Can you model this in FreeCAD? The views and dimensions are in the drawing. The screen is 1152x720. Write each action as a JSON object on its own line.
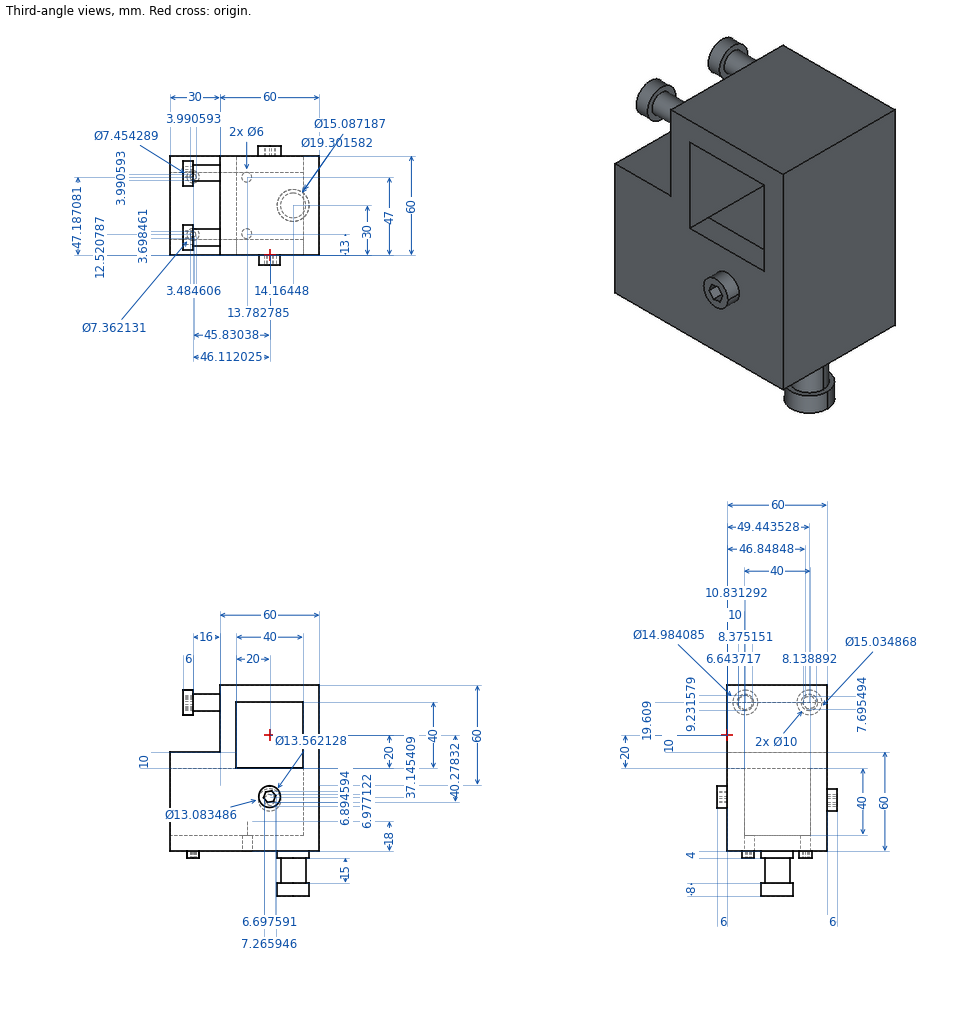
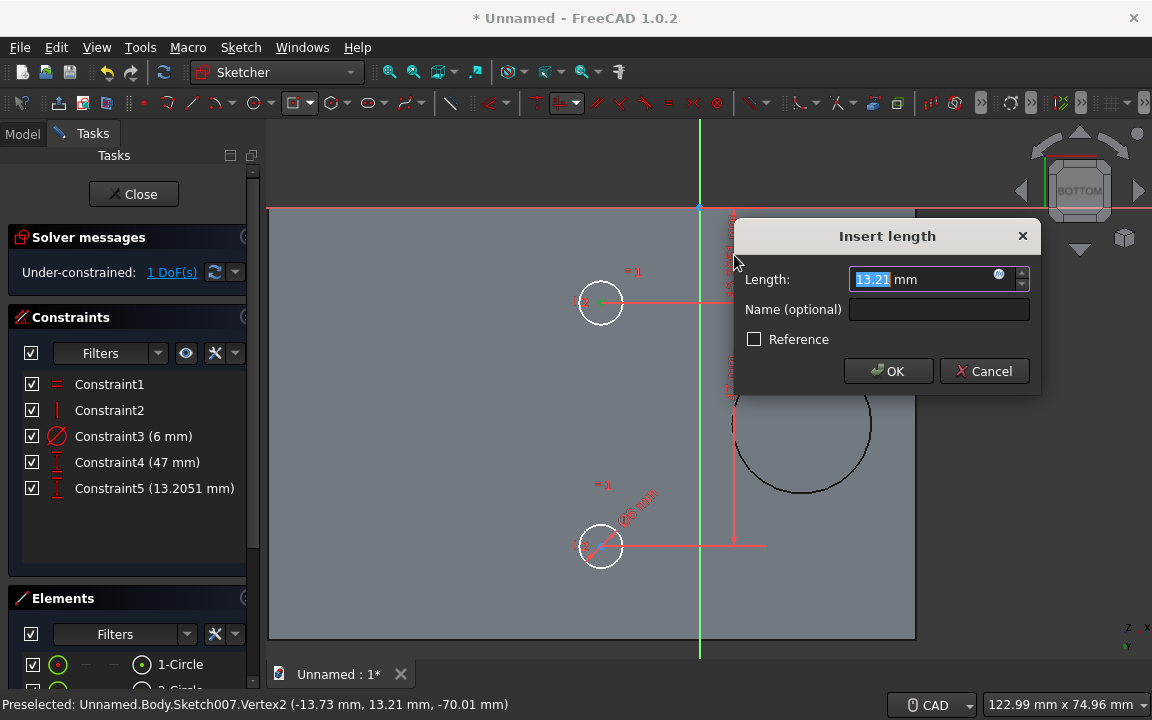
{"action": "type", "text": "13"}
{"action": "key", "text": "Return"}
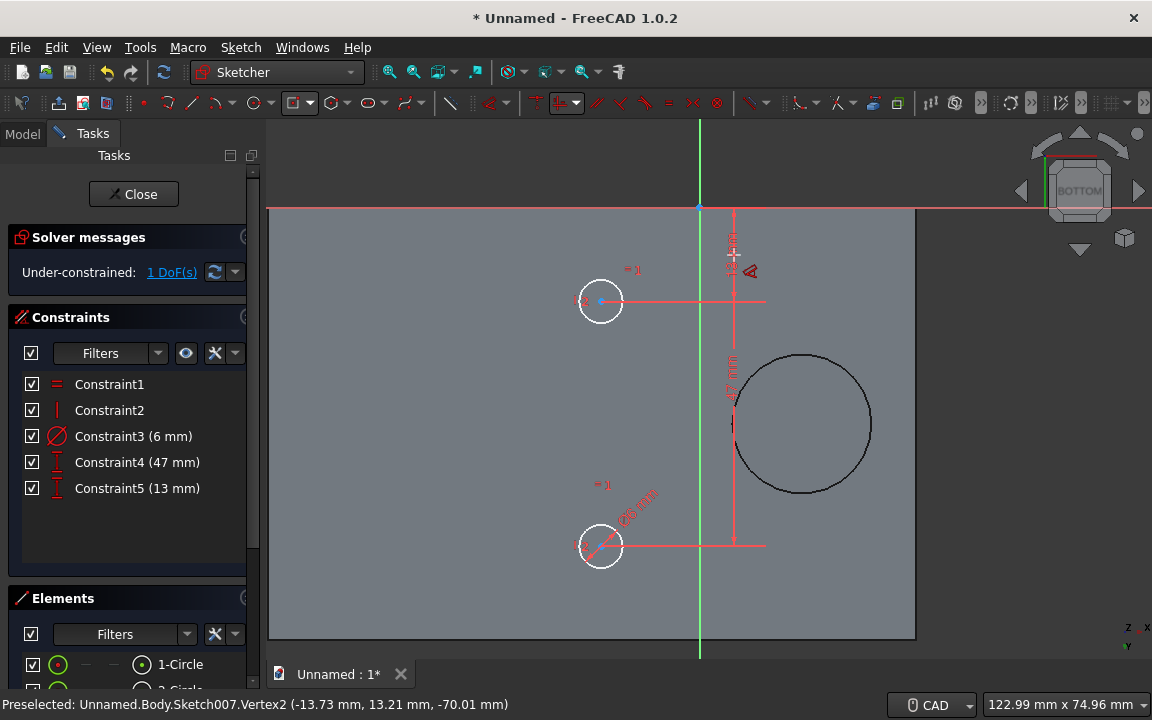
{"action": "left_click", "coordinate": [601, 546]}
{"action": "left_click", "coordinate": [650, 174]}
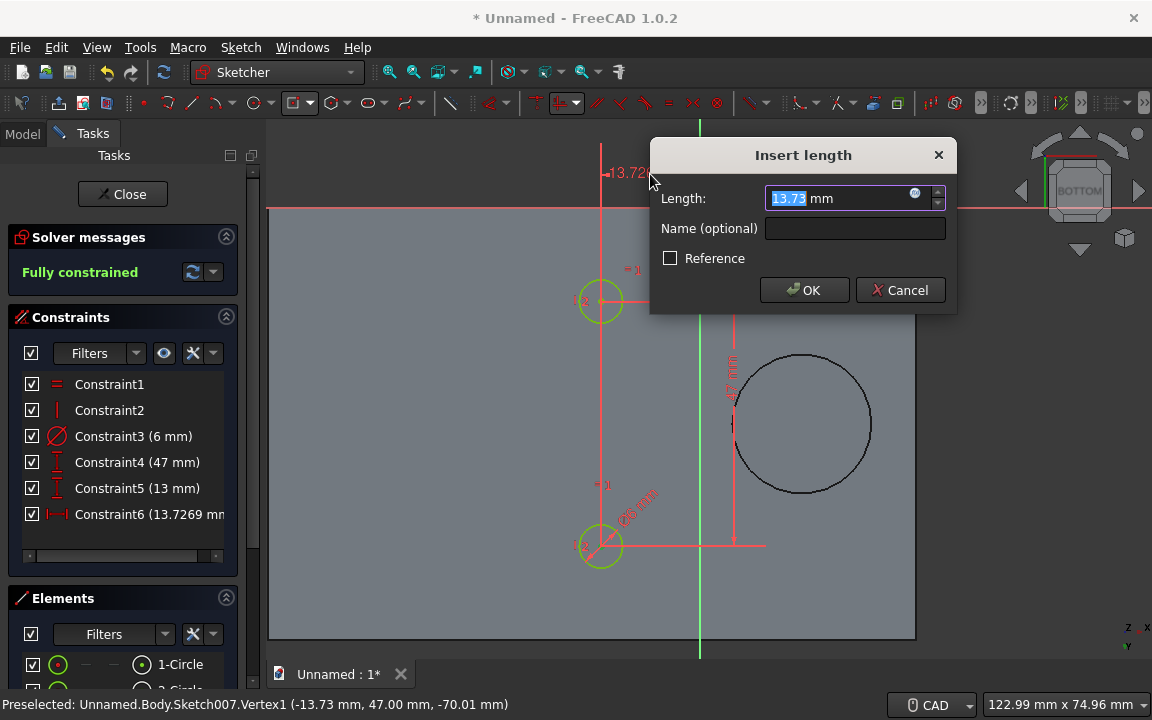
{"action": "type", "text": "13.782785"}
{"action": "key", "text": "Return"}
{"action": "key", "text": "Escape"}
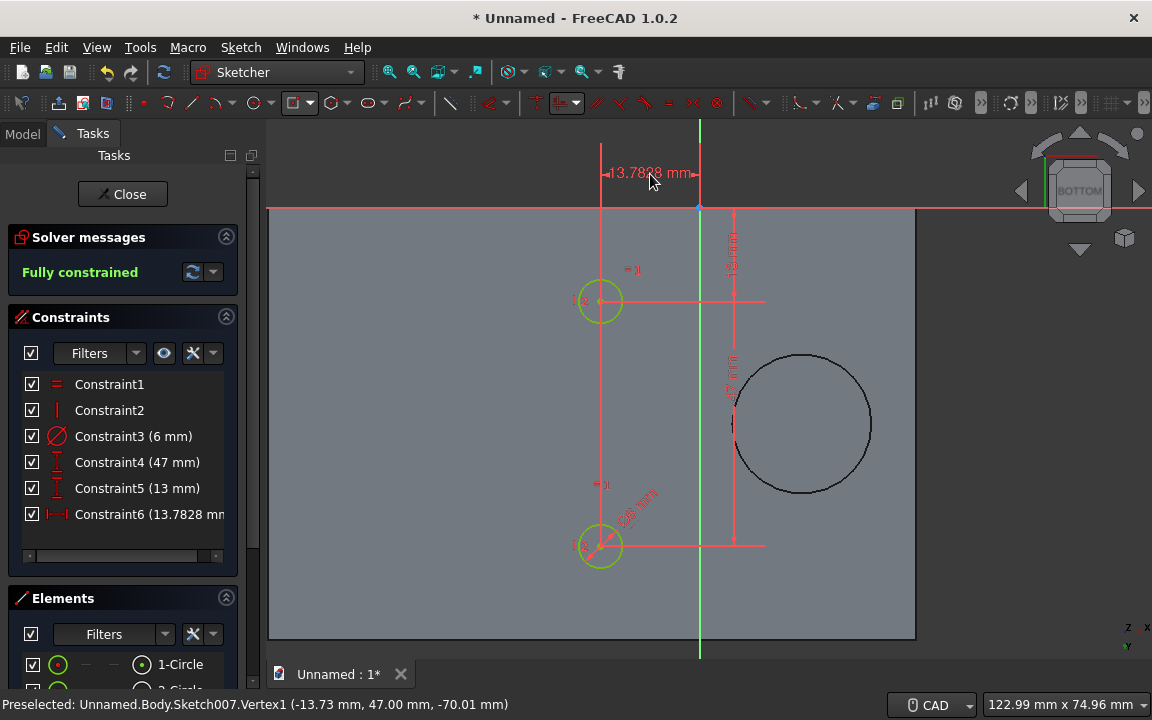
{"action": "left_click", "coordinate": [123, 194]}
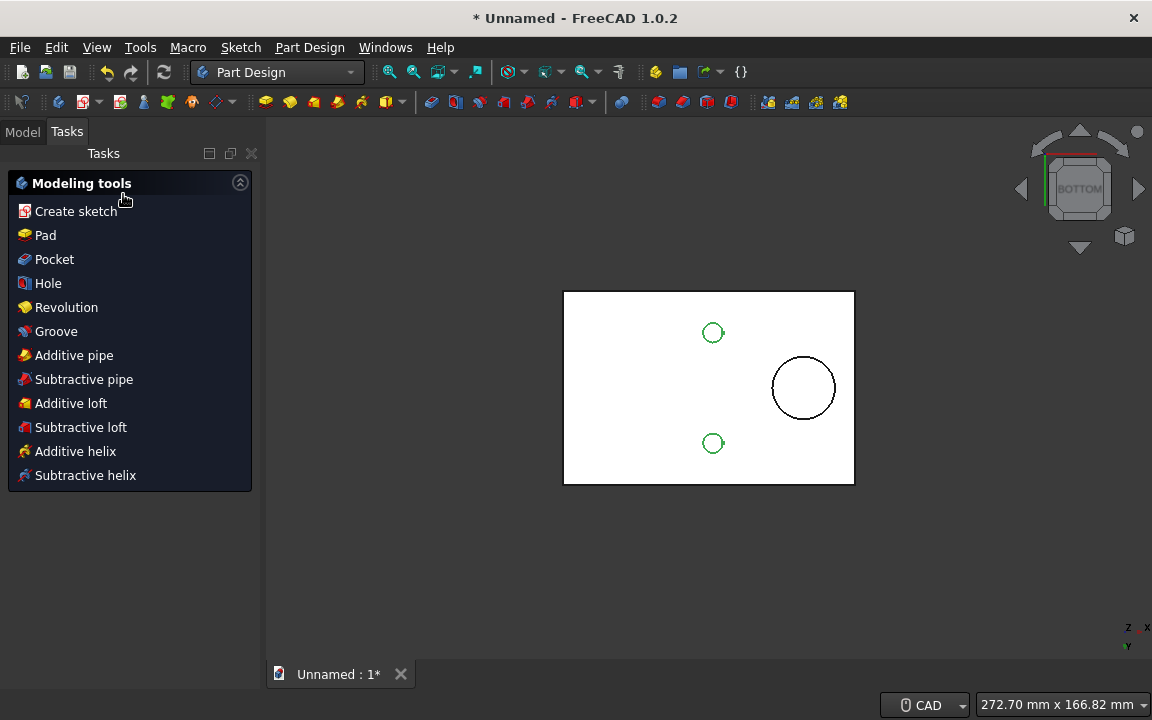
{"action": "left_click", "coordinate": [432, 102]}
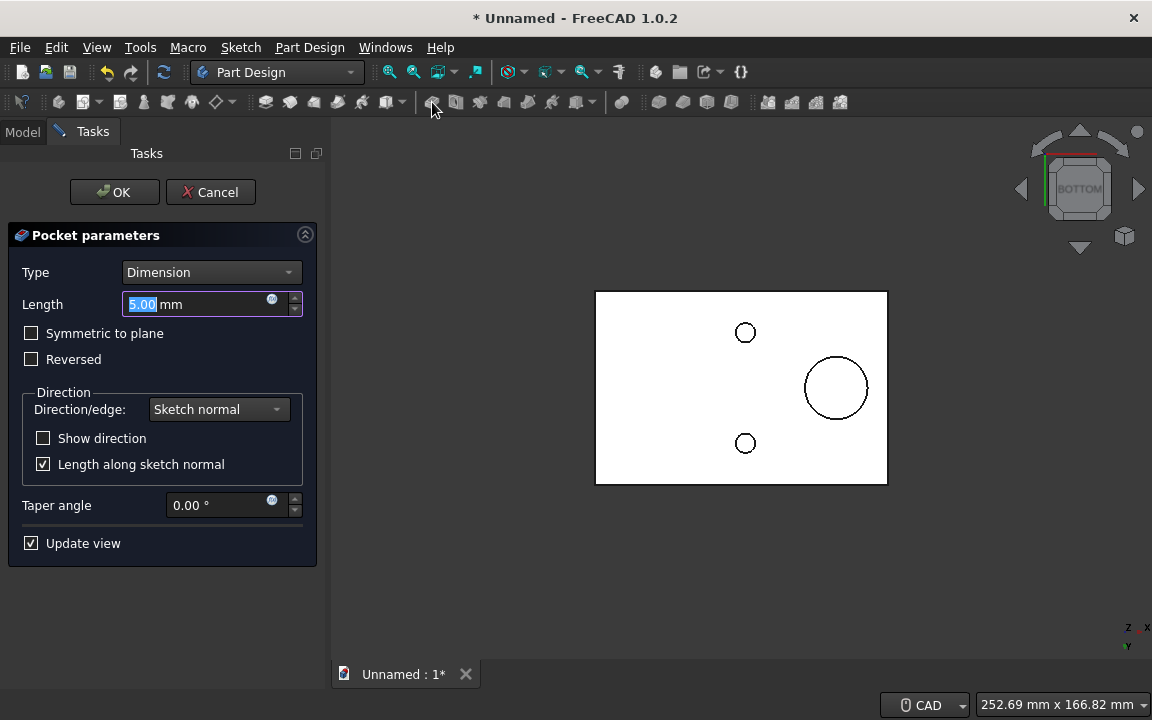
{"action": "type", "text": "18"}
{"action": "key", "text": "Tab"}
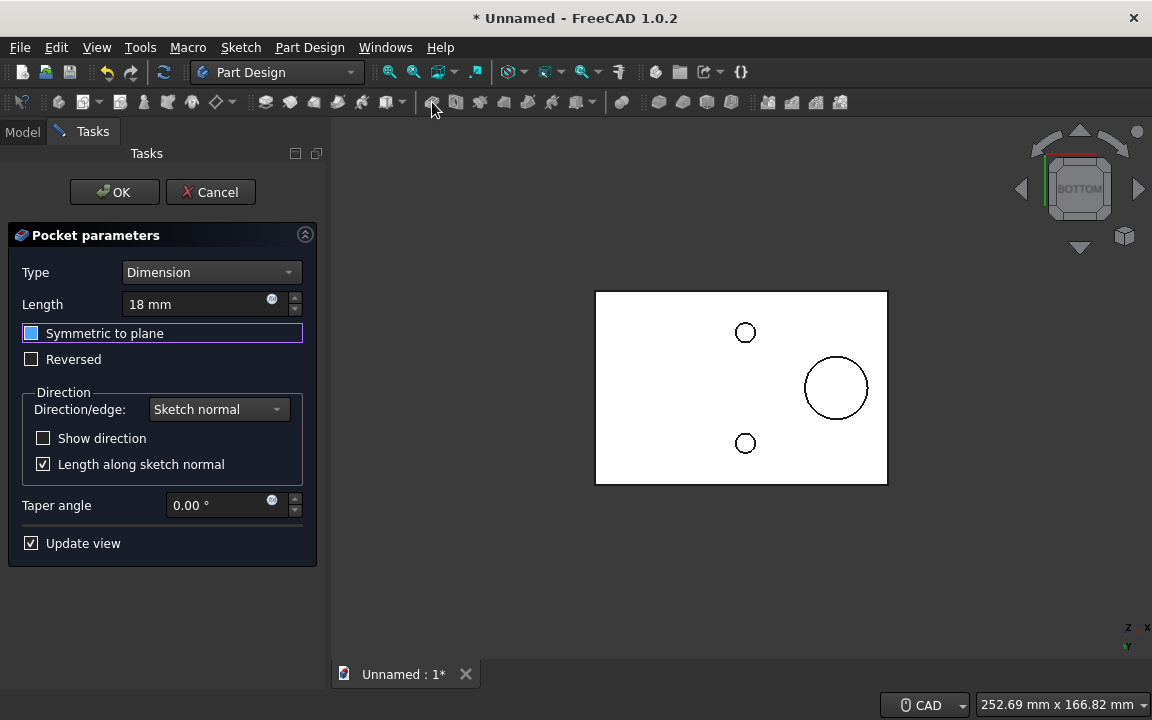
{"action": "left_click", "coordinate": [115, 192]}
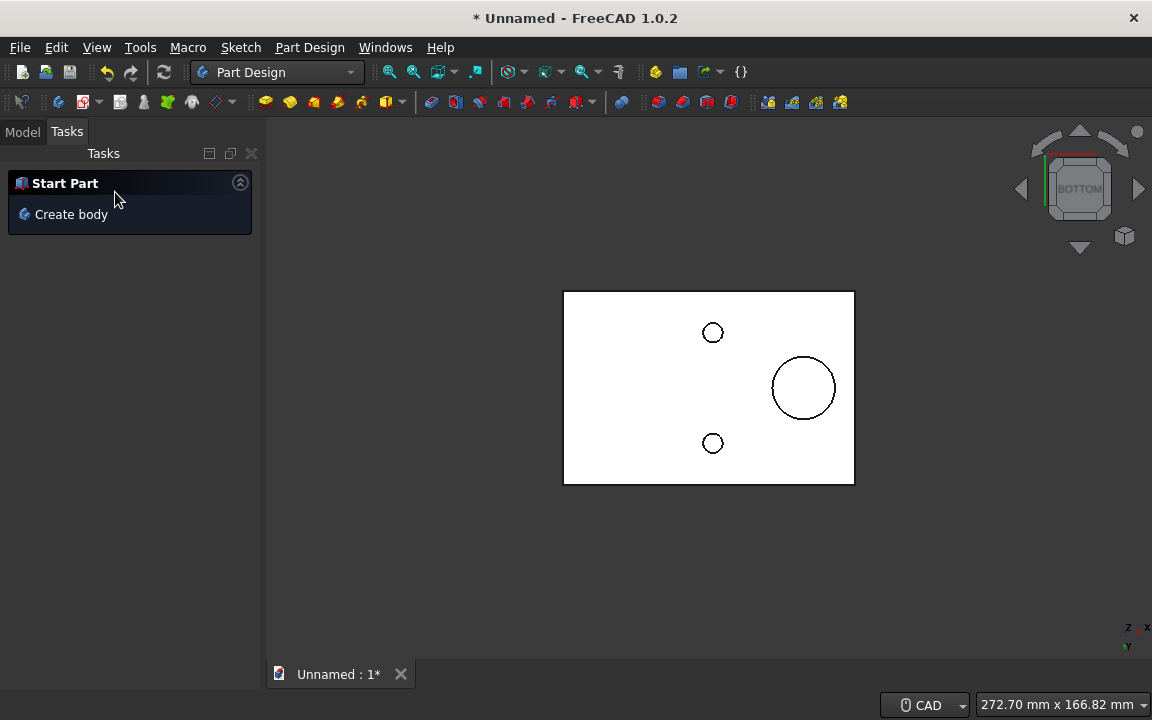
{"action": "left_click", "coordinate": [390, 72]}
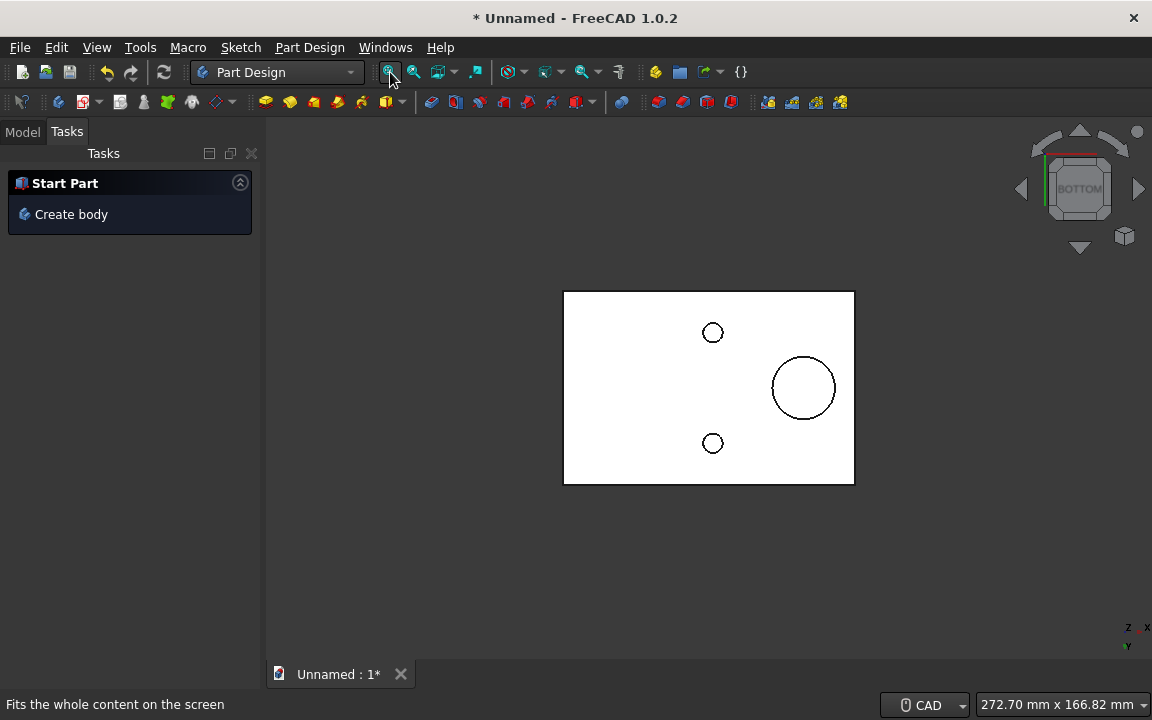
{"action": "left_click", "coordinate": [625, 415]}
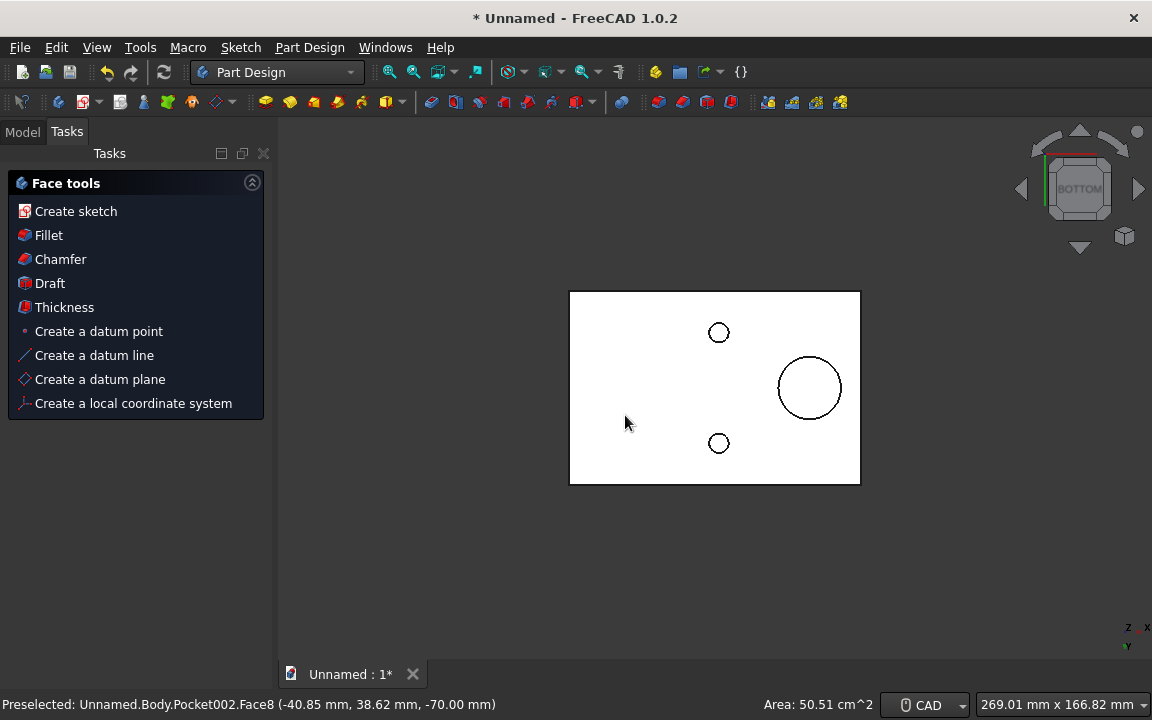
{"action": "left_click", "coordinate": [84, 102]}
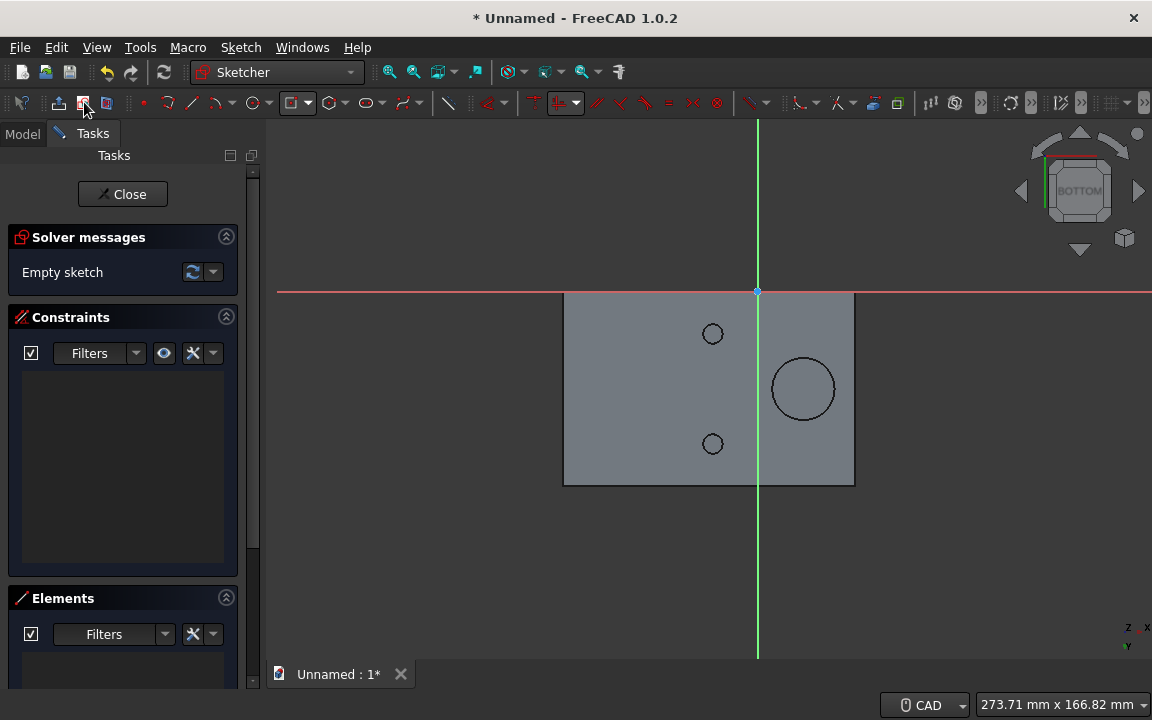
{"action": "scroll", "coordinate": [707, 362], "scroll_direction": "up", "scroll_amount": 4}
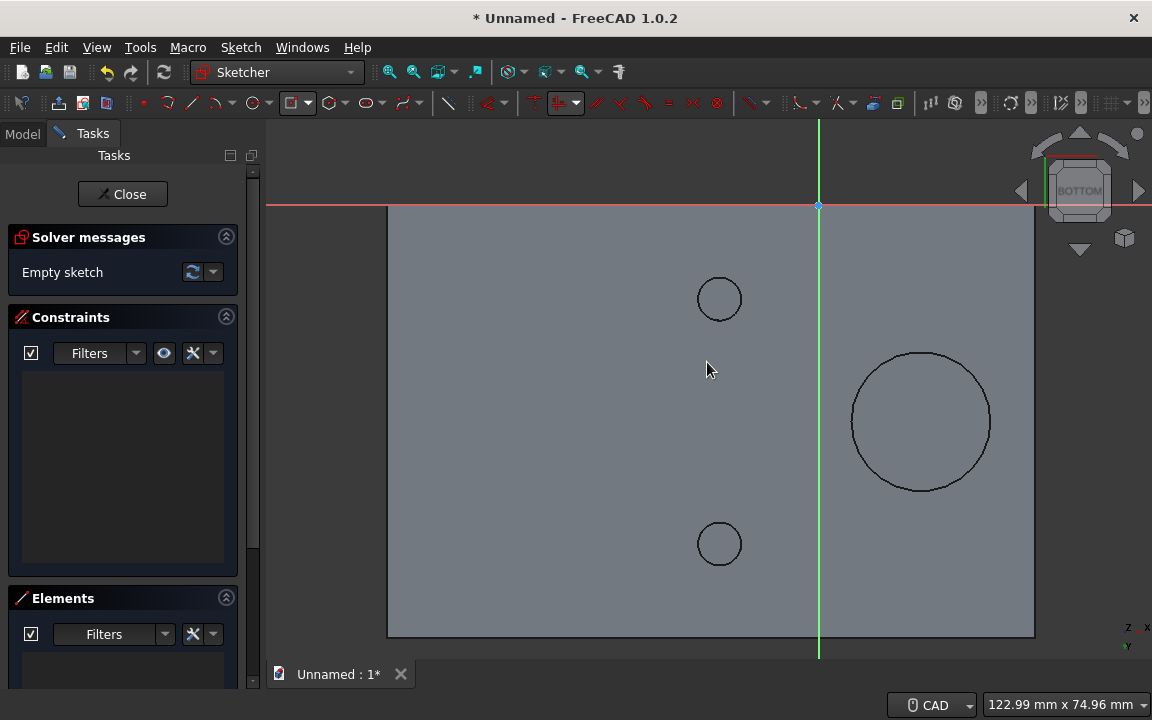
{"action": "left_click", "coordinate": [330, 104]}